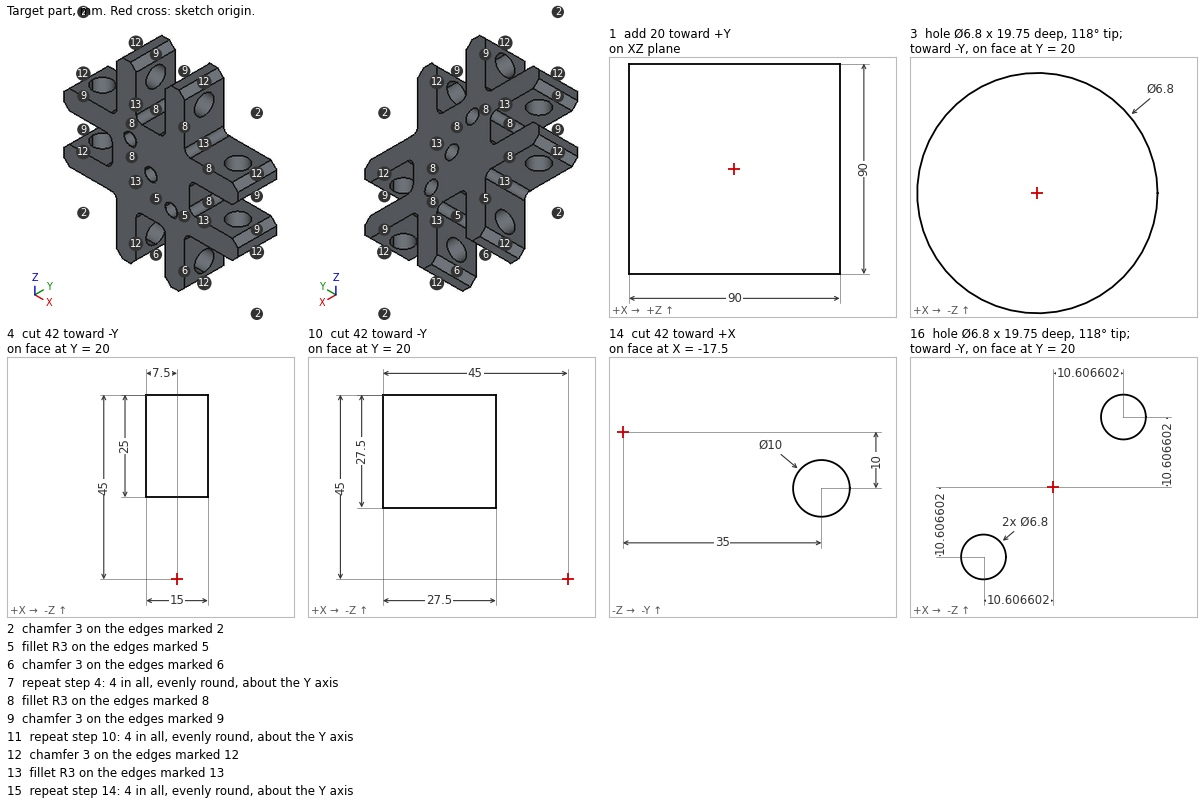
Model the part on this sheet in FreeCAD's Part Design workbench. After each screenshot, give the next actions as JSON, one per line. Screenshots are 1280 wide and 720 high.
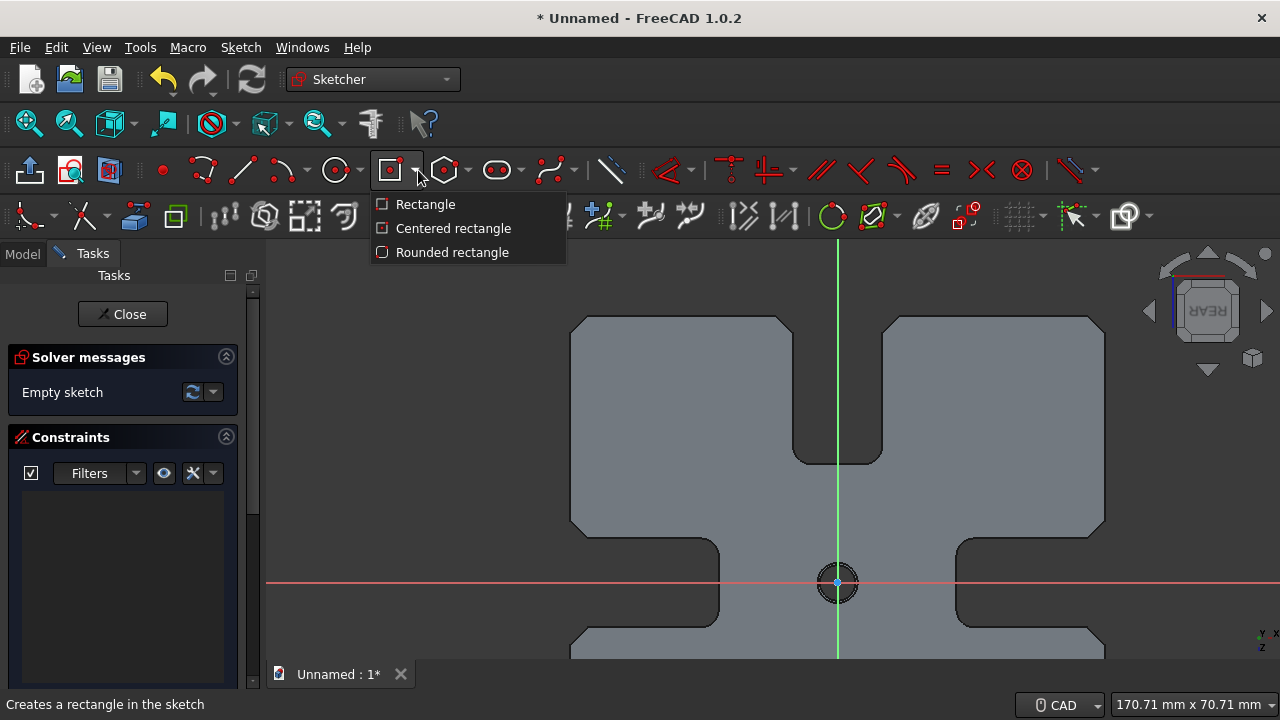
{"action": "left_click", "coordinate": [468, 204]}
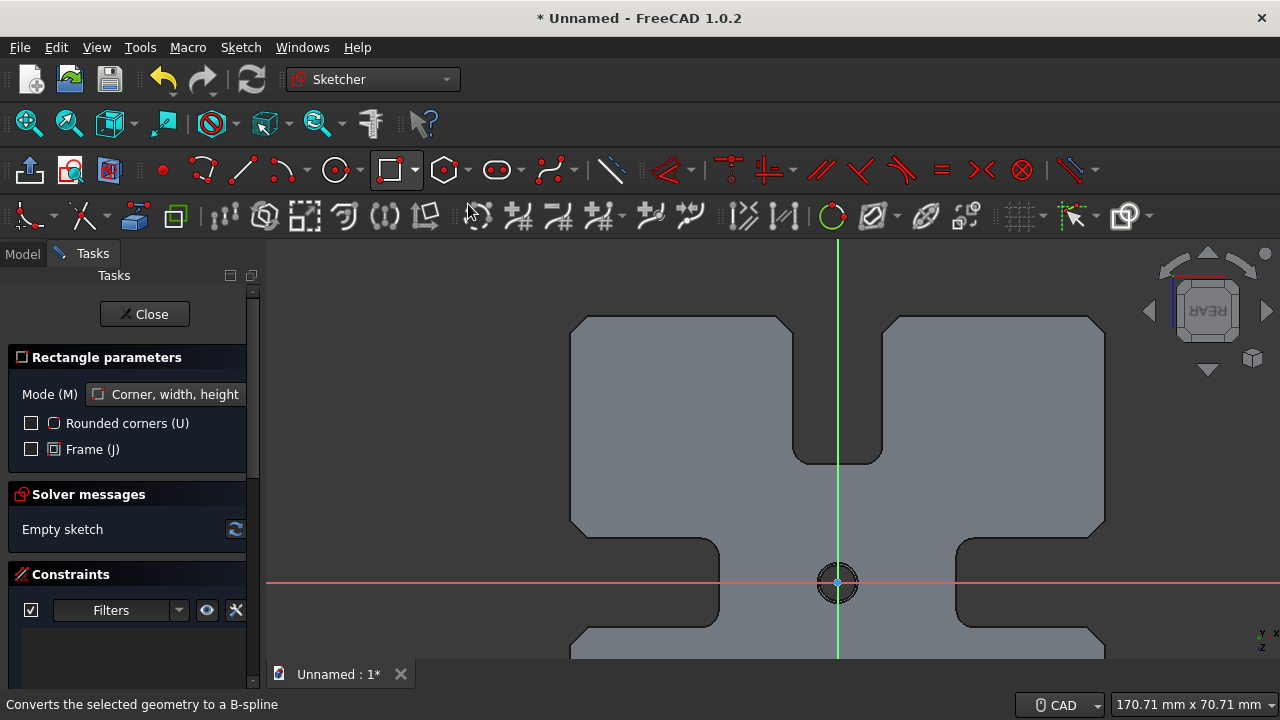
{"action": "left_click", "coordinate": [570, 316]}
{"action": "left_click", "coordinate": [734, 479]}
{"action": "key", "text": "Escape"}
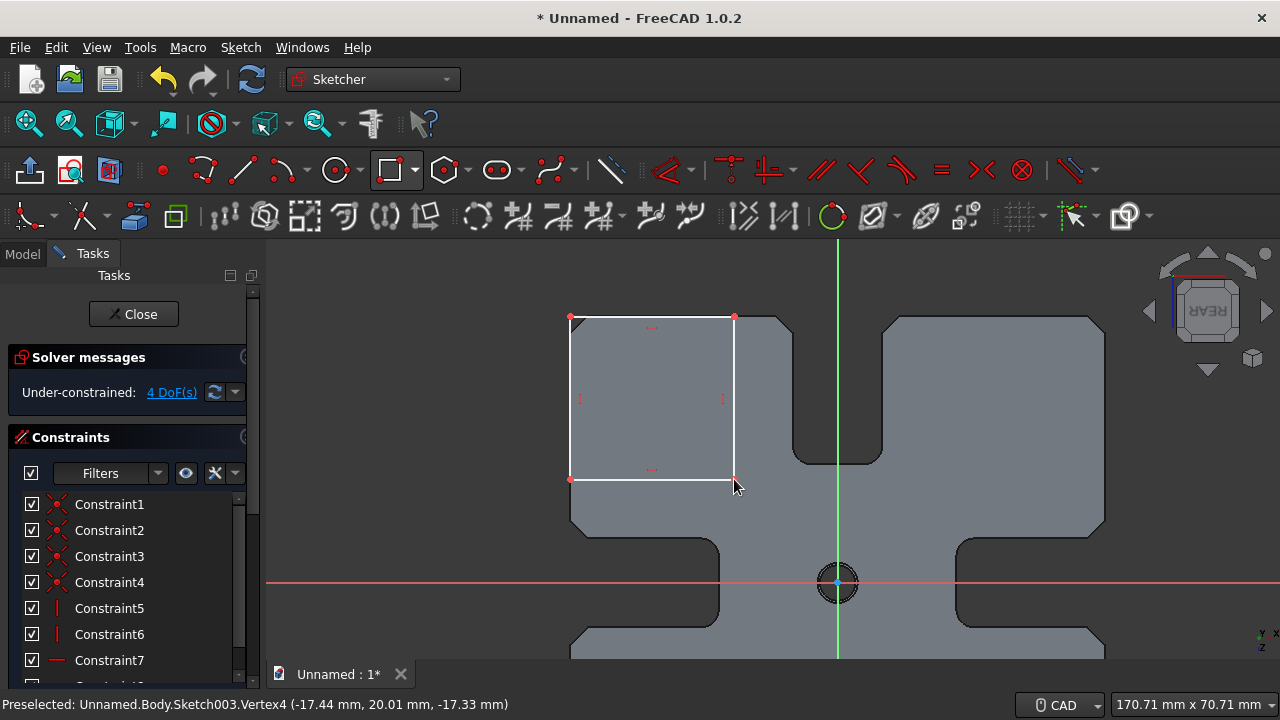
{"action": "left_click", "coordinate": [666, 170]}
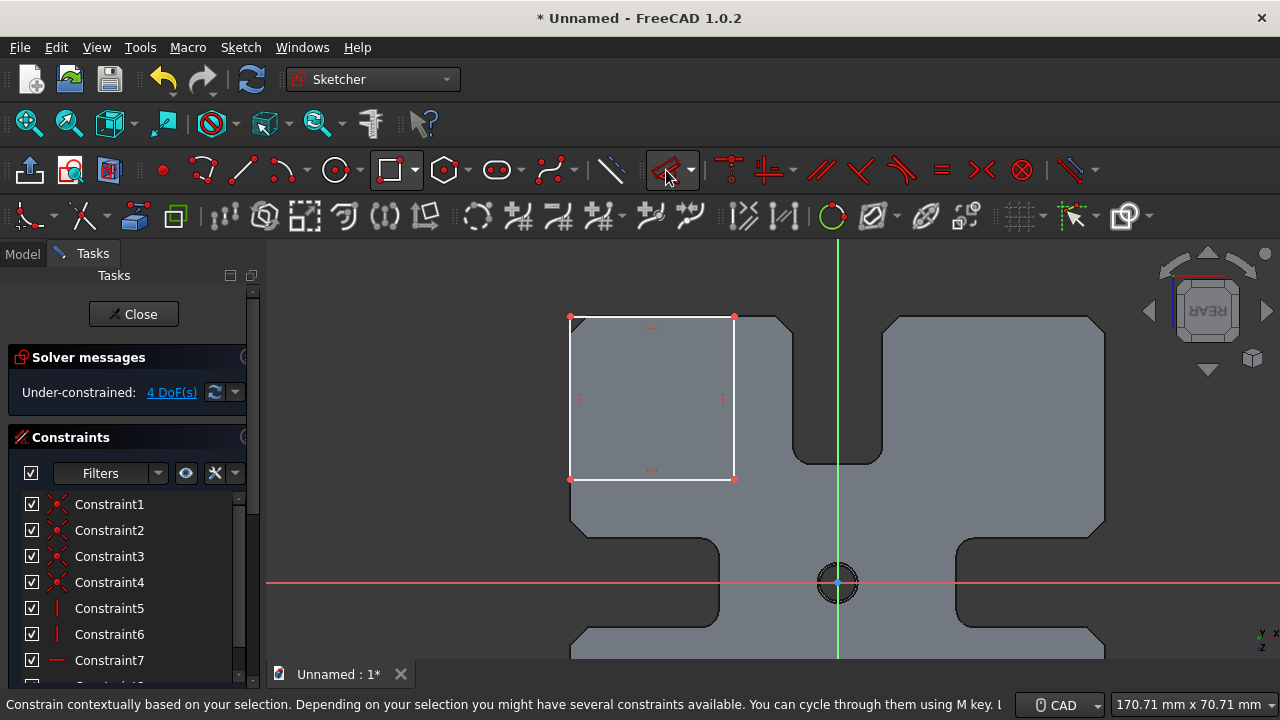
{"action": "left_click", "coordinate": [570, 317]}
{"action": "left_click", "coordinate": [704, 617]}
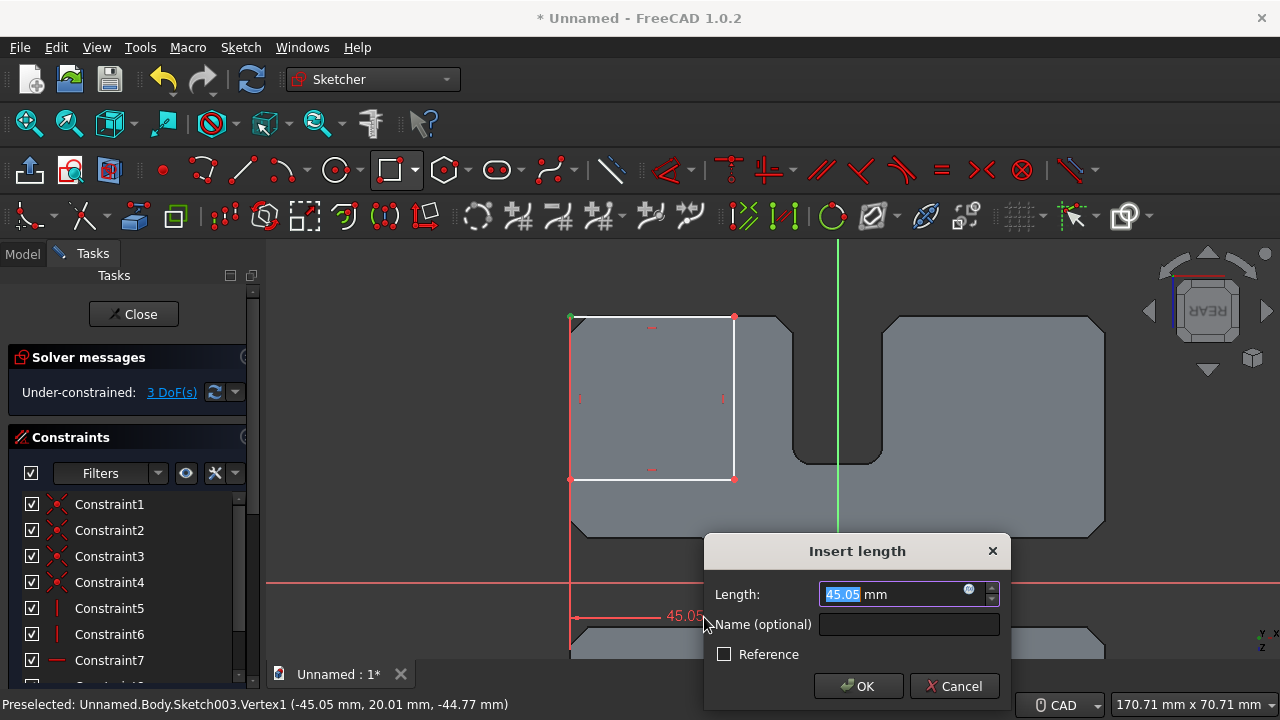
{"action": "type", "text": "45"}
{"action": "key", "text": "Return"}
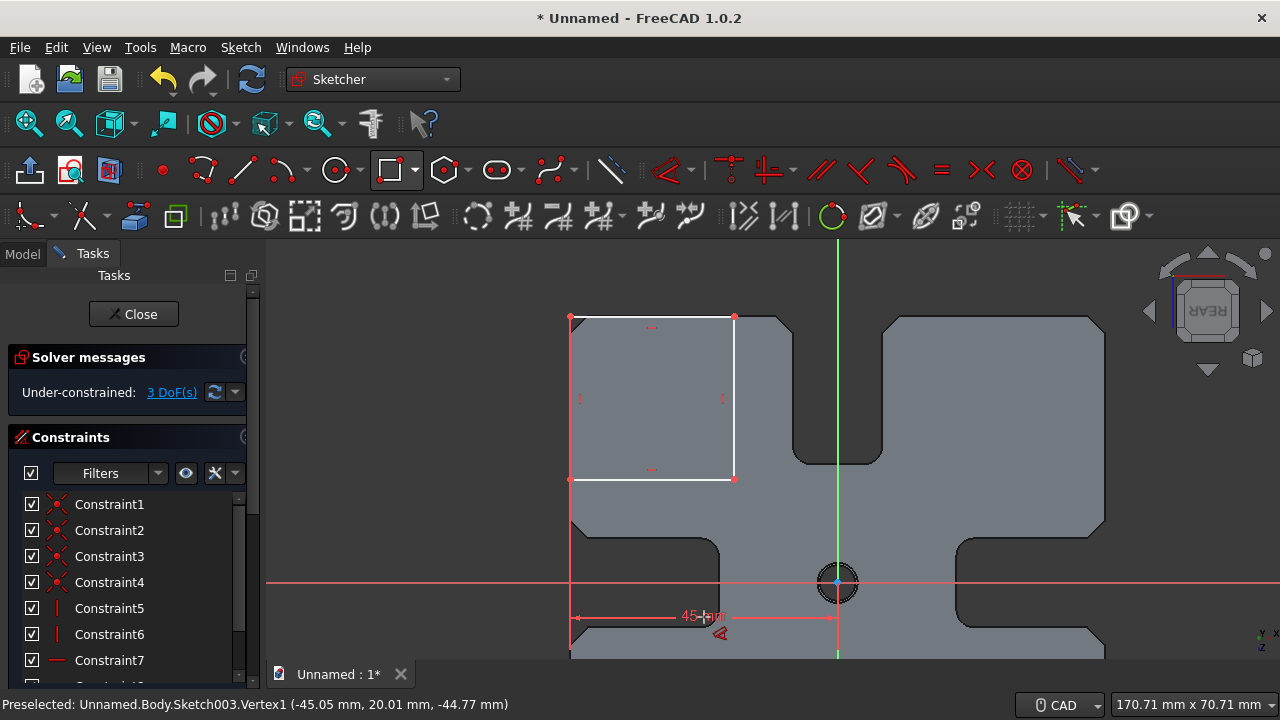
{"action": "left_click", "coordinate": [570, 317]}
{"action": "left_click", "coordinate": [872, 450]}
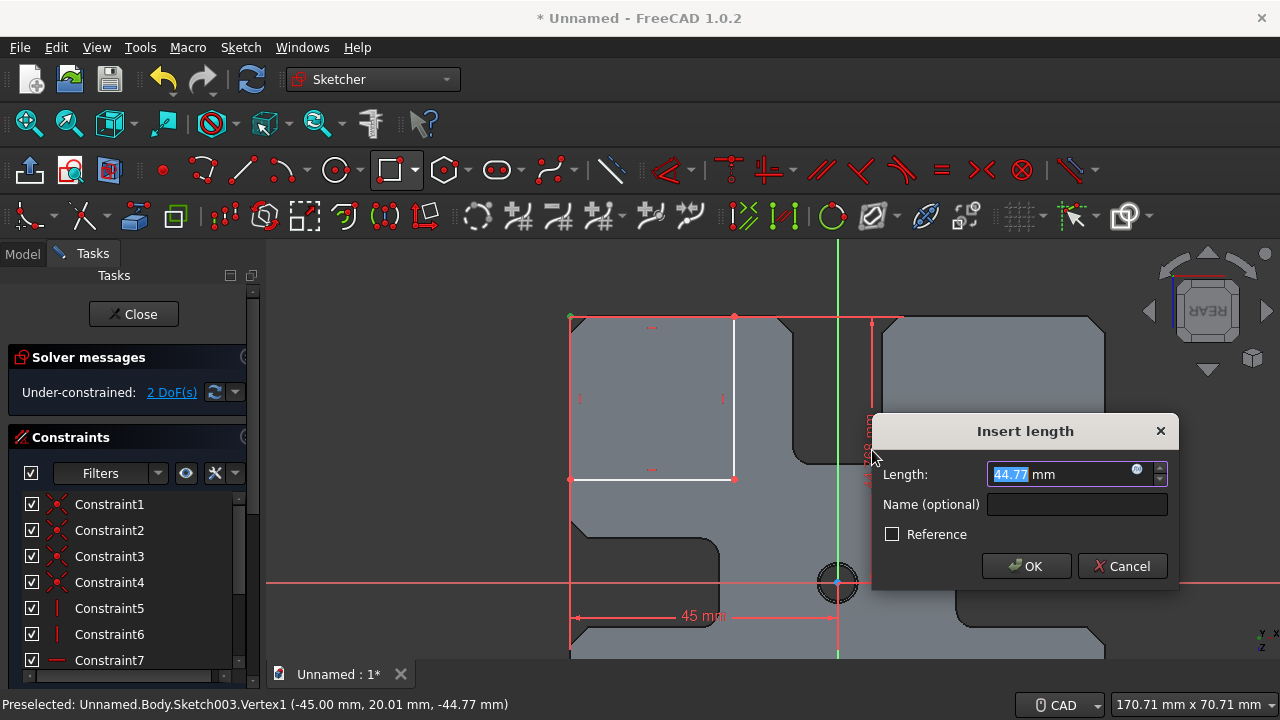
{"action": "type", "text": "45"}
{"action": "key", "text": "Return"}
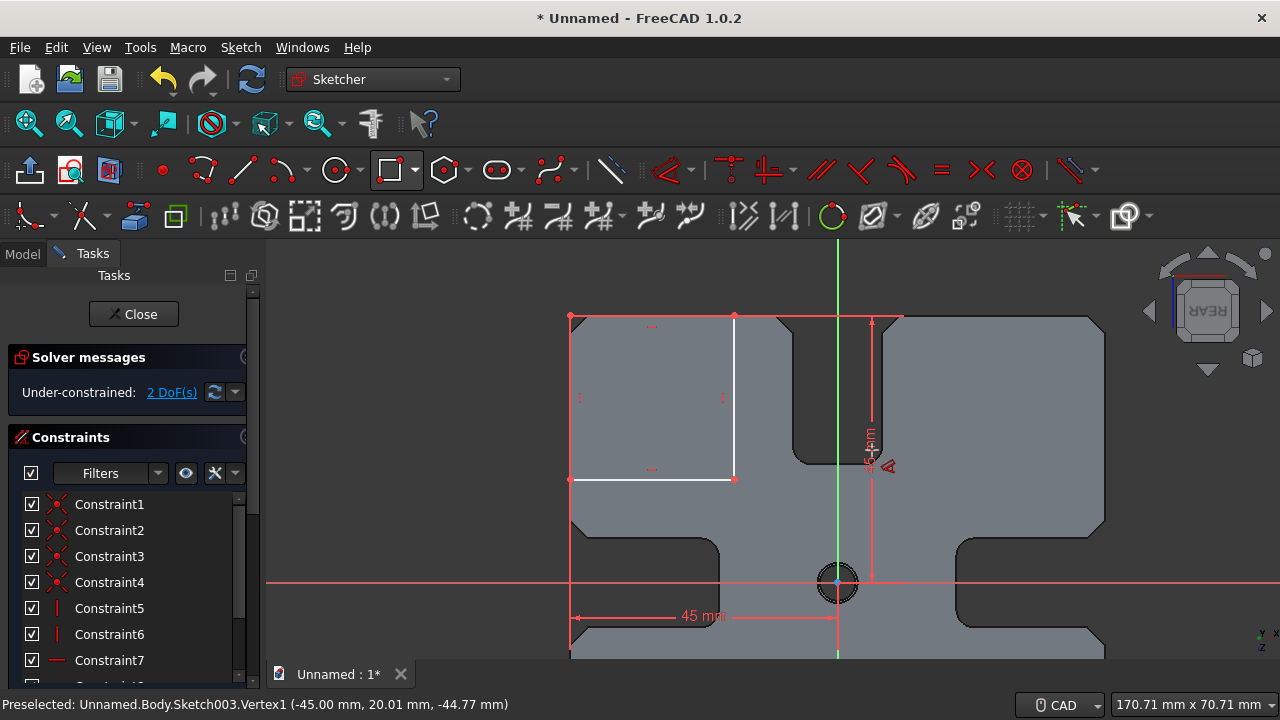
{"action": "left_click", "coordinate": [570, 365]}
{"action": "left_click", "coordinate": [536, 398]}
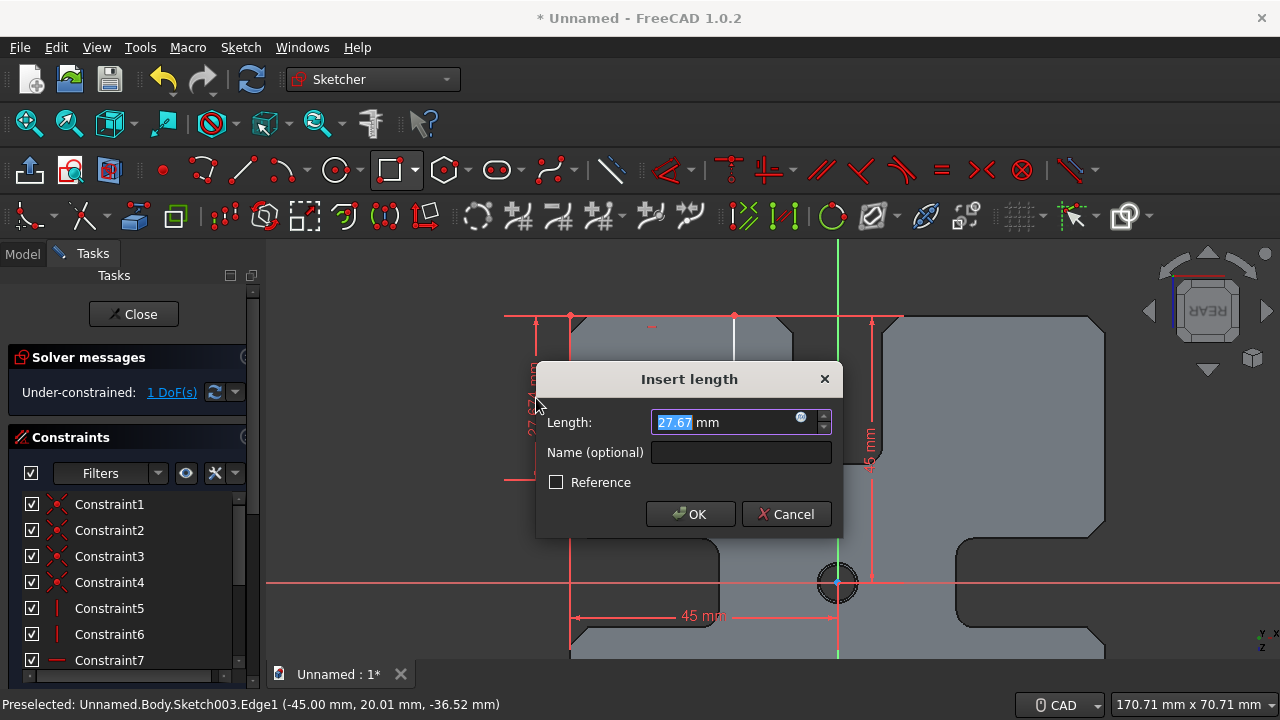
{"action": "type", "text": "27.5"}
{"action": "key", "text": "Return"}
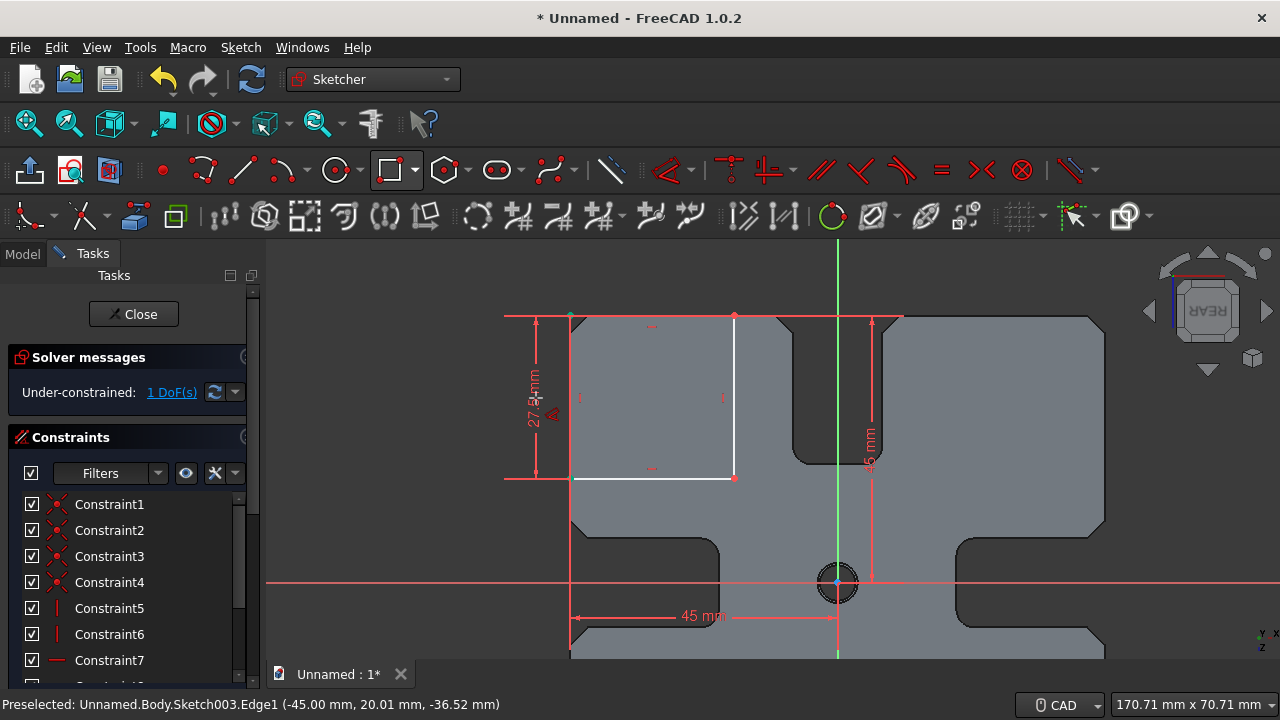
{"action": "left_click", "coordinate": [619, 479]}
{"action": "left_click", "coordinate": [652, 513]}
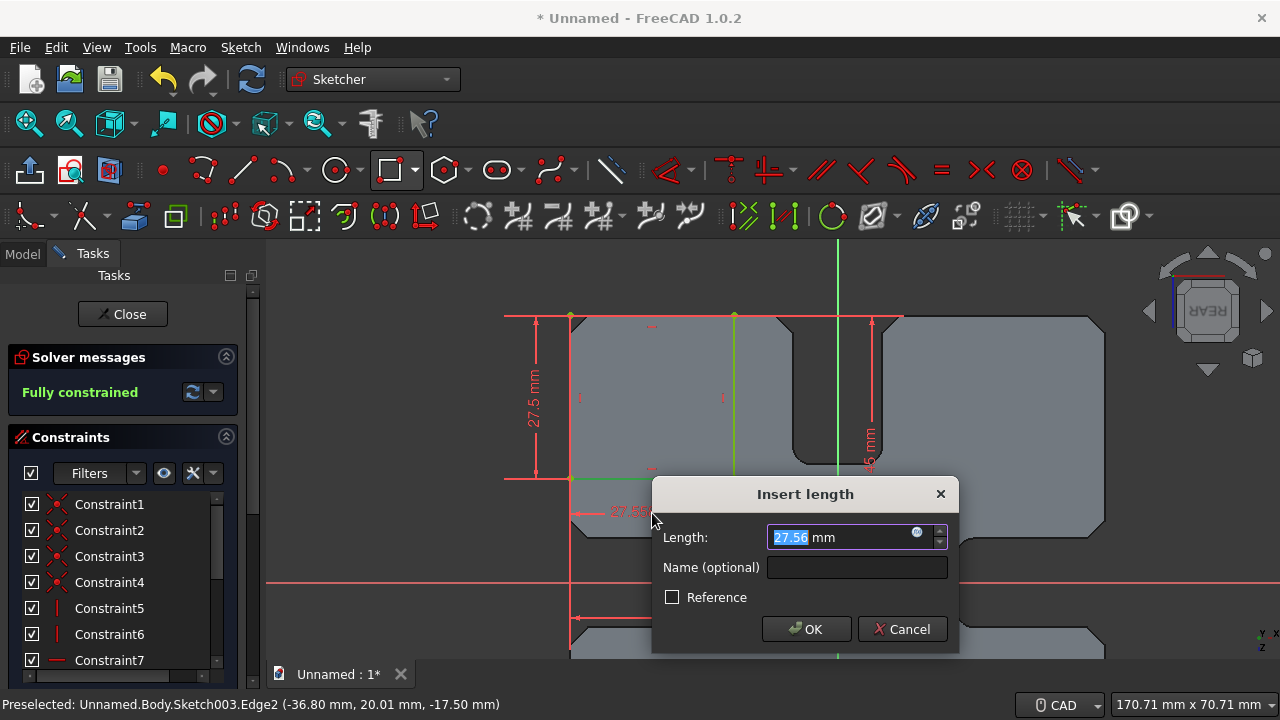
{"action": "type", "text": "27.5"}
{"action": "key", "text": "Return"}
{"action": "key", "text": "Escape"}